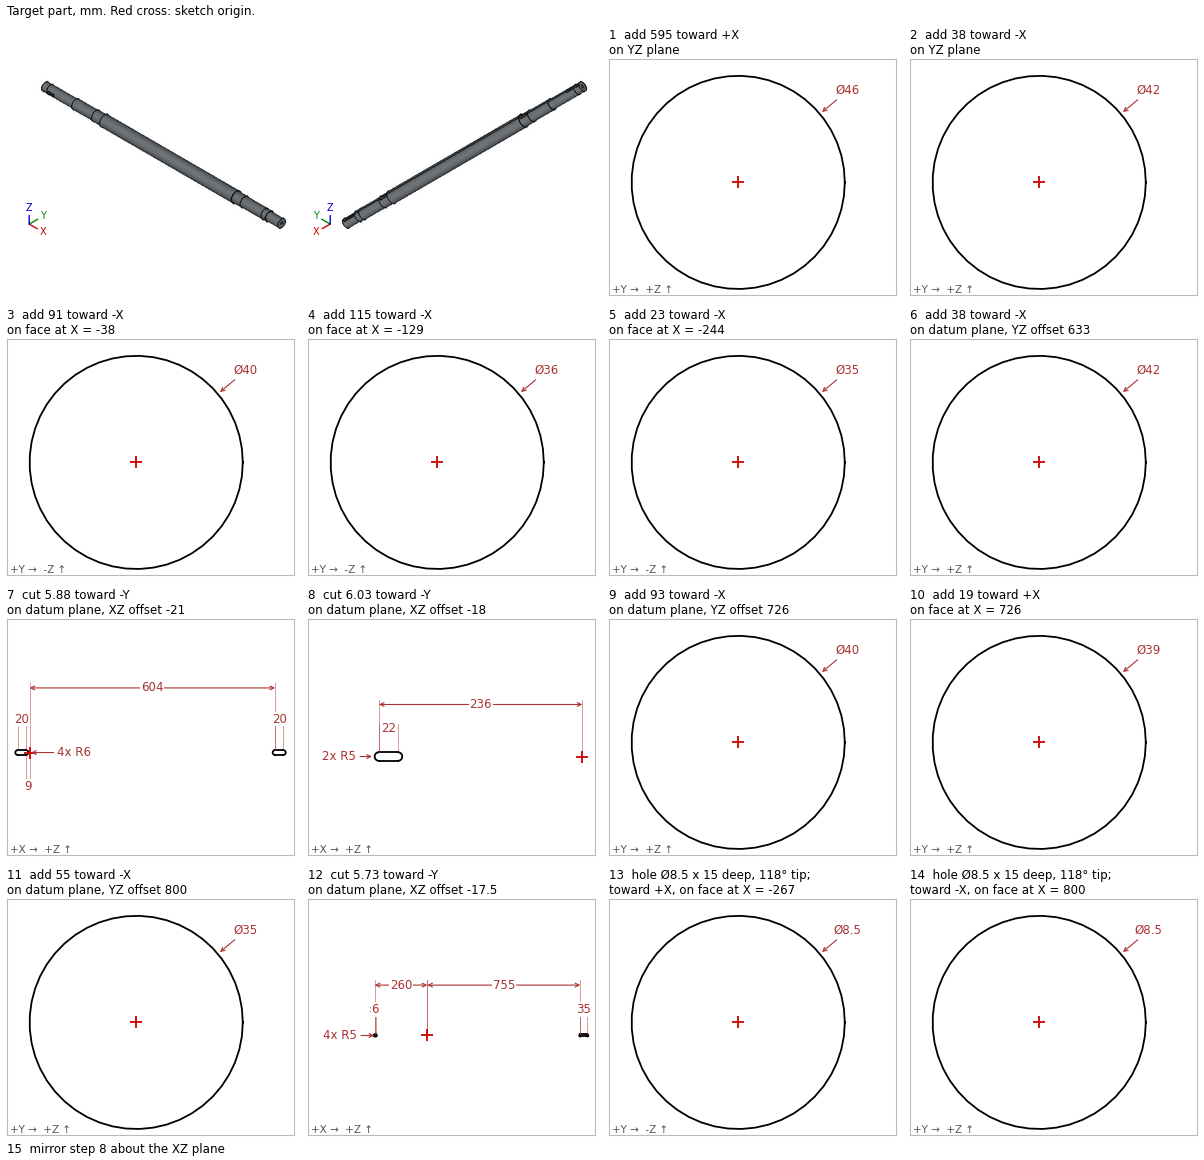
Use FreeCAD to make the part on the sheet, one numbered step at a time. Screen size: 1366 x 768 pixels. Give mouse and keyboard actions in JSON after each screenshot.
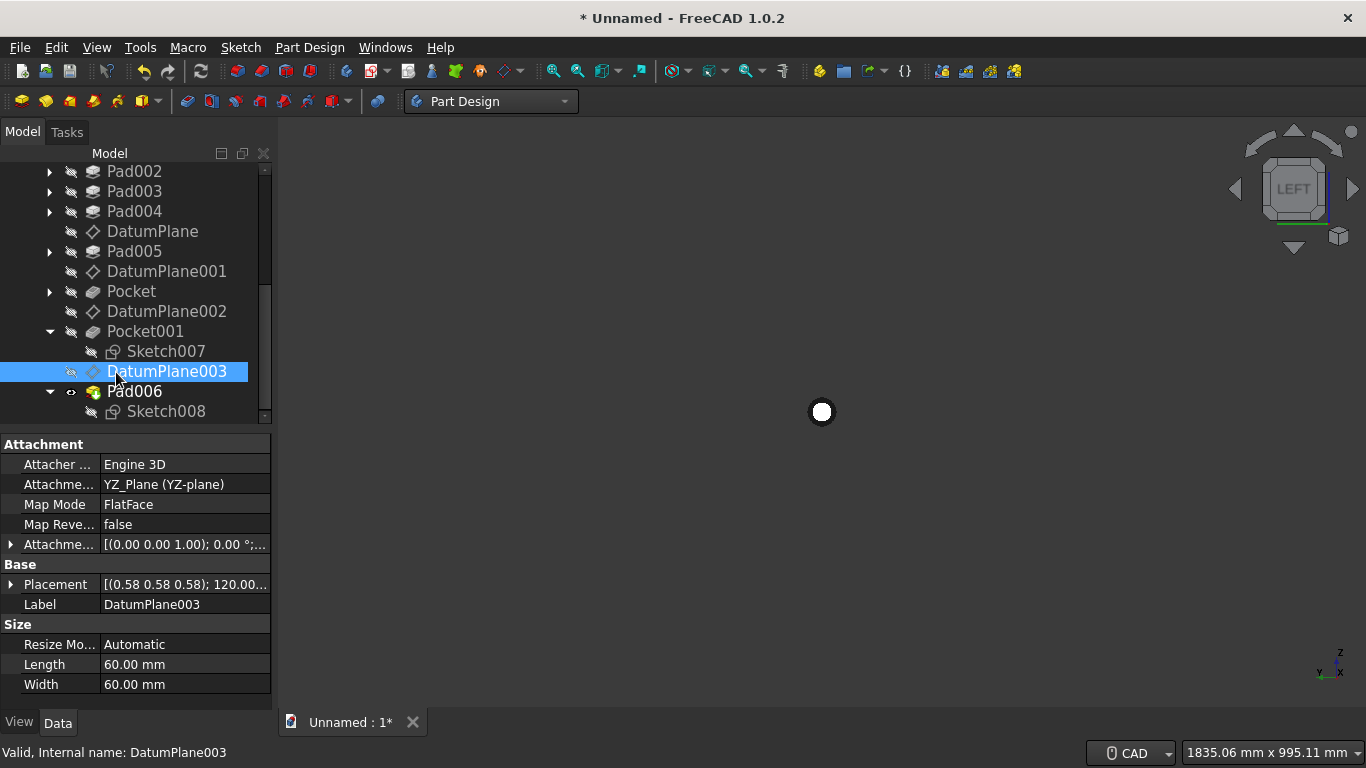
{"action": "key", "text": "0"}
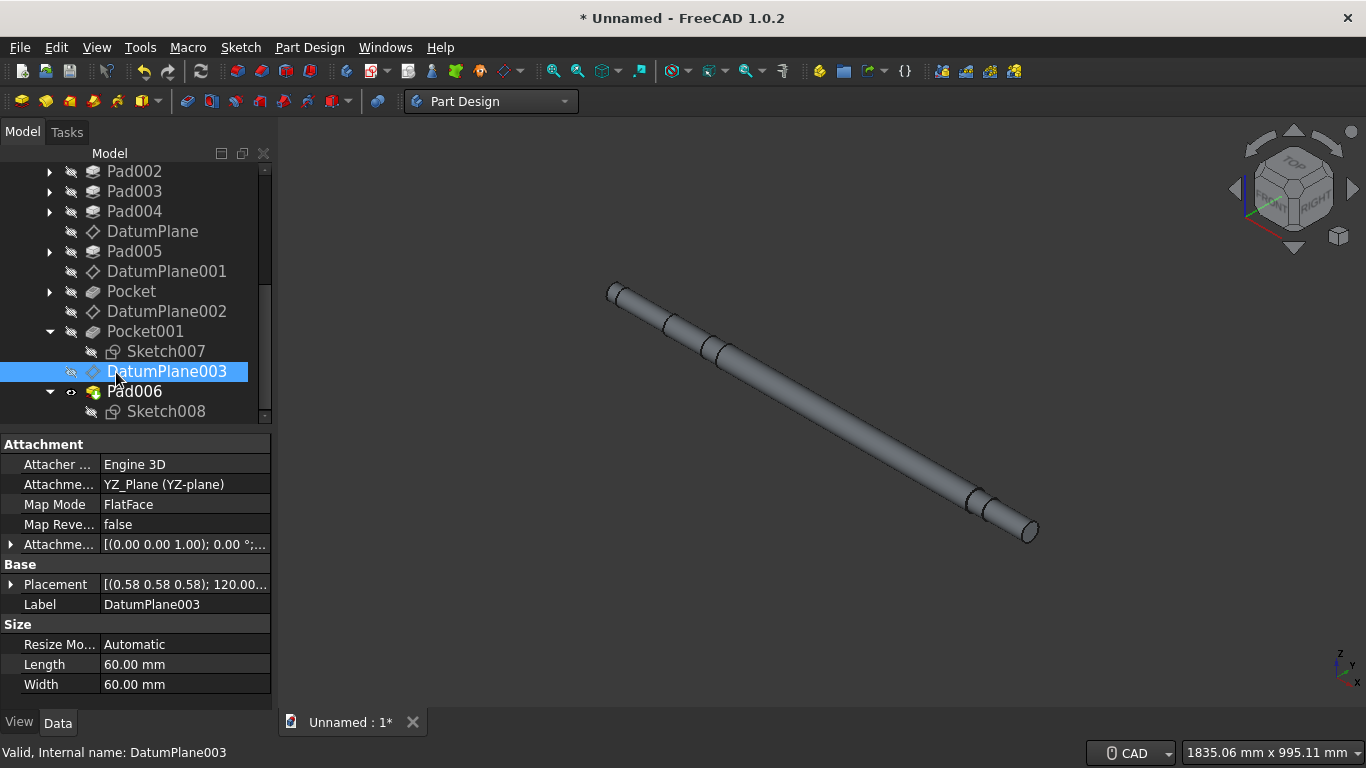
{"action": "key", "text": "3"}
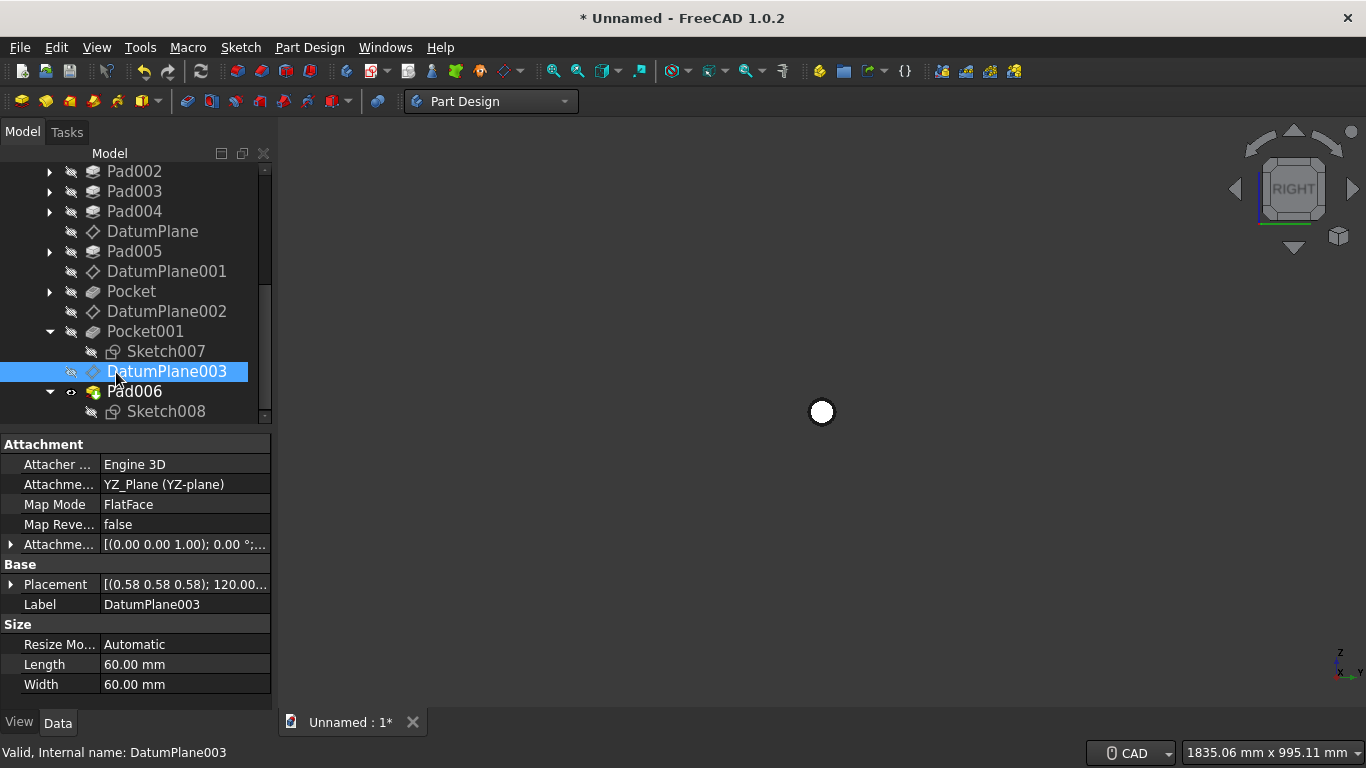
{"action": "left_click", "coordinate": [554, 72]}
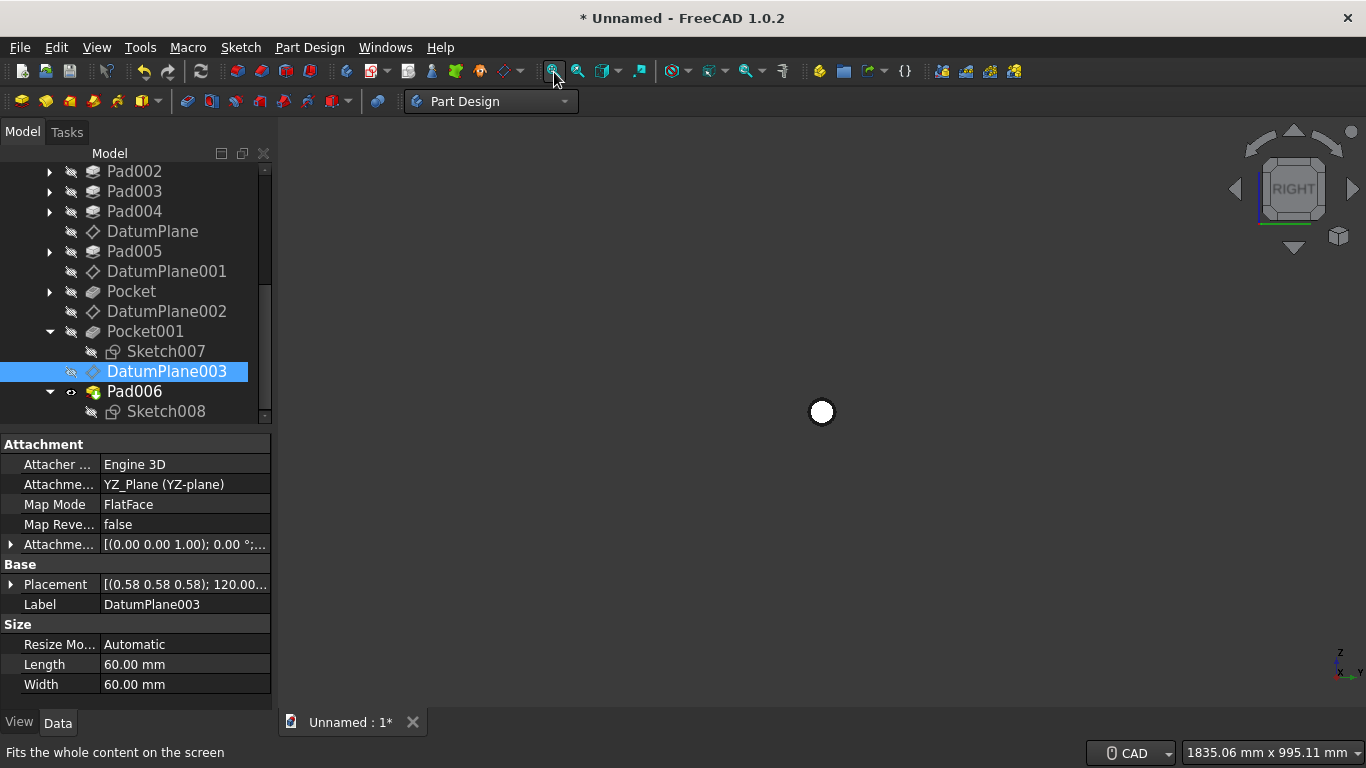
{"action": "left_click", "coordinate": [822, 411]}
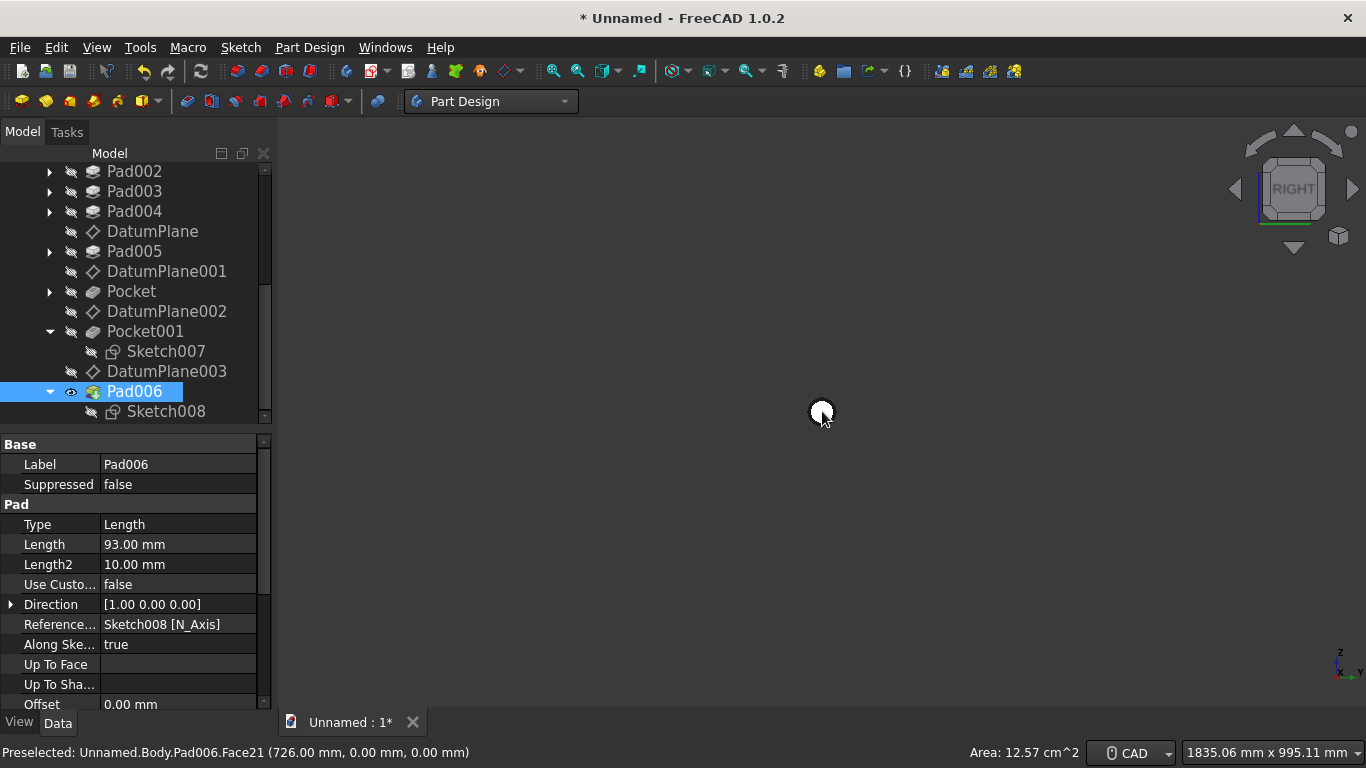
{"action": "left_click", "coordinate": [372, 72]}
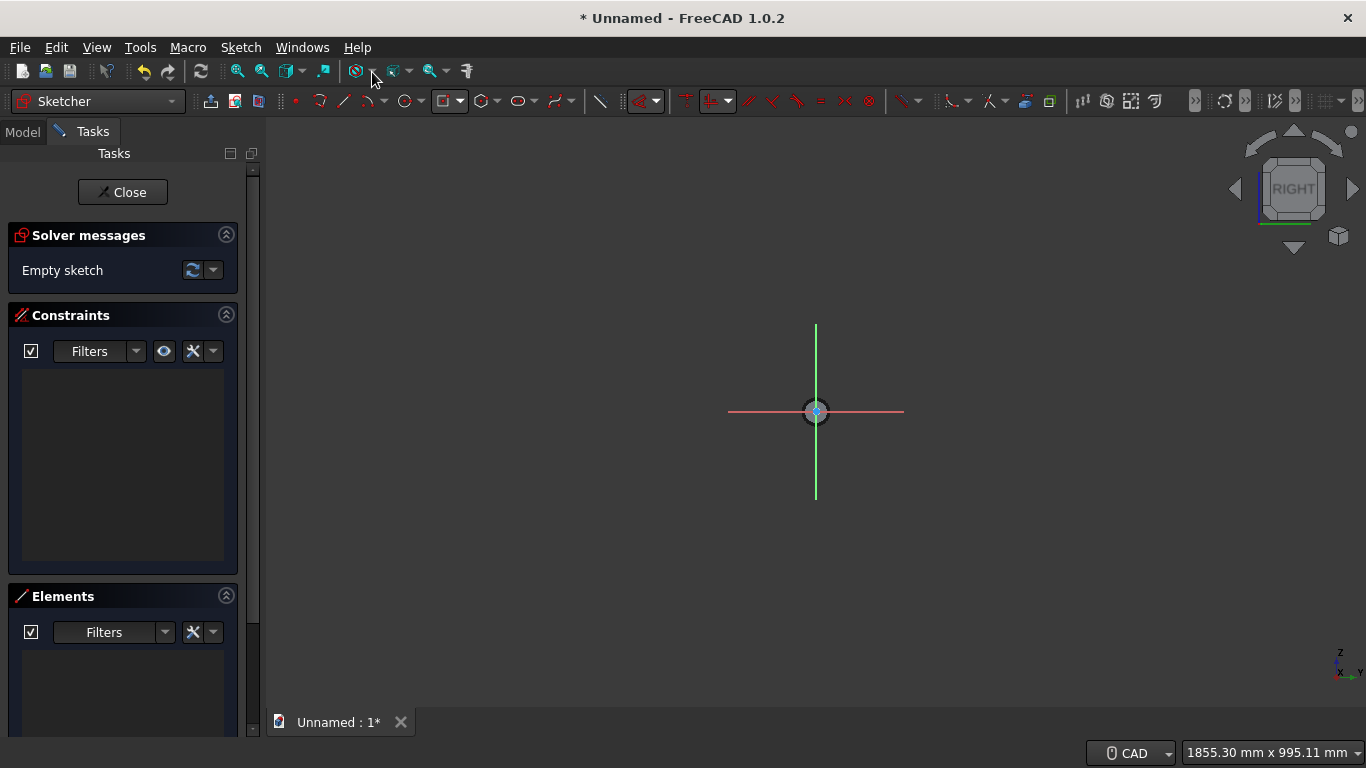
{"action": "scroll", "coordinate": [820, 412], "scroll_direction": "up", "scroll_amount": 14}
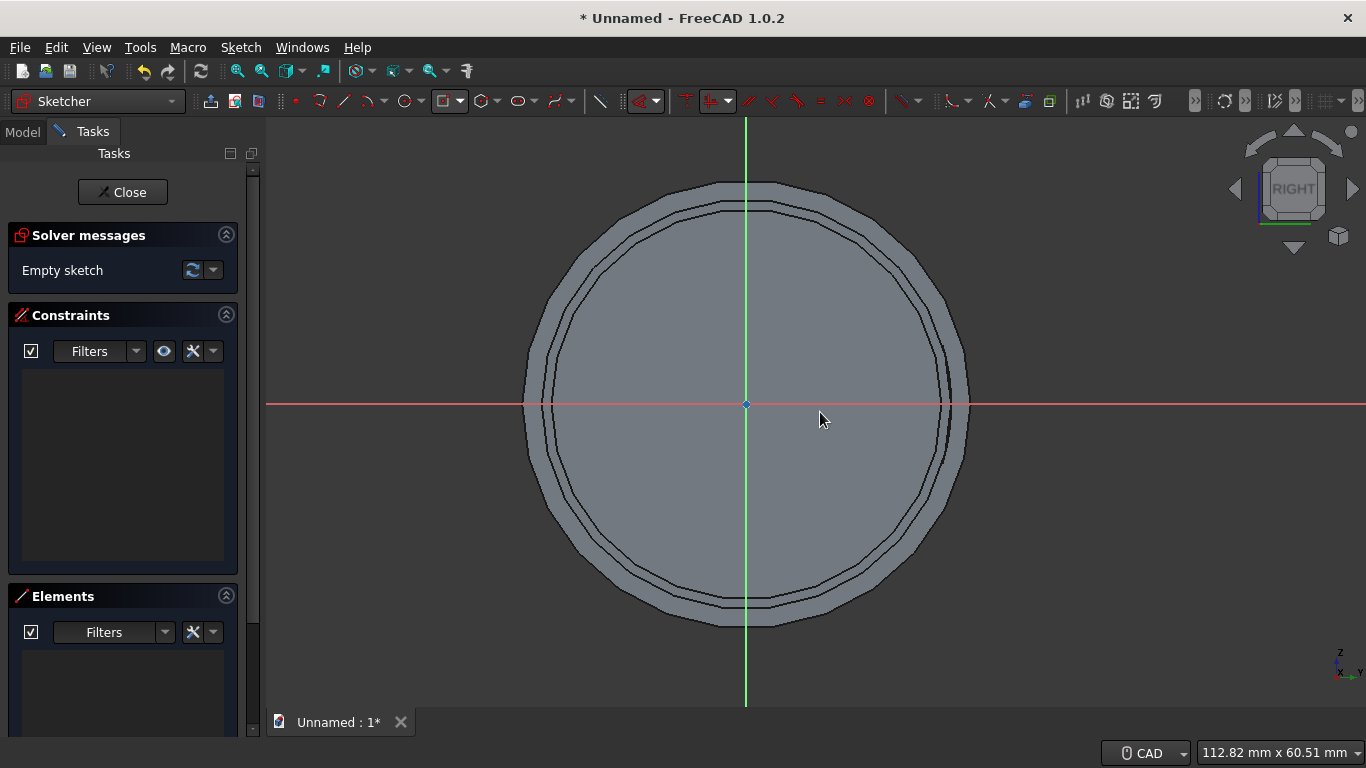
{"action": "key", "text": "g c"}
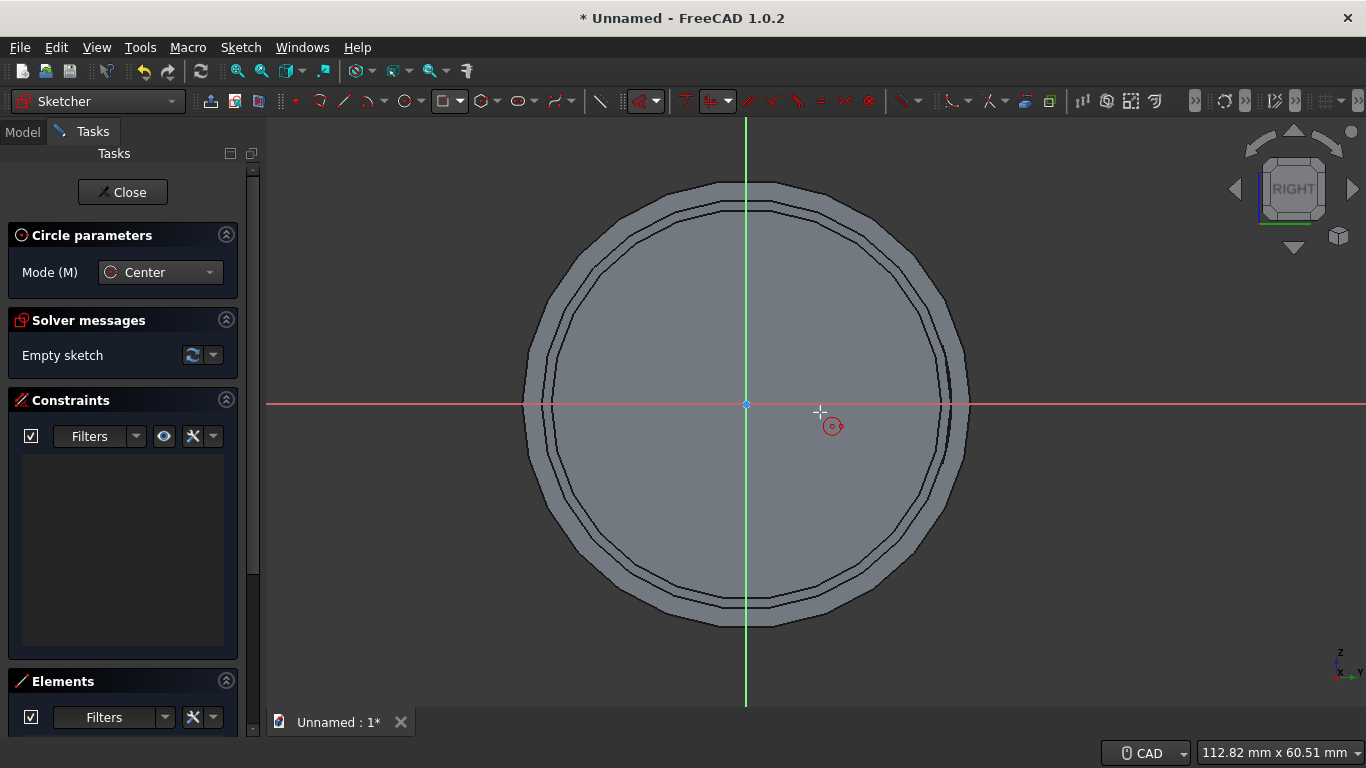
{"action": "left_click", "coordinate": [746, 404]}
{"action": "mouse_move", "coordinate": [881, 270]}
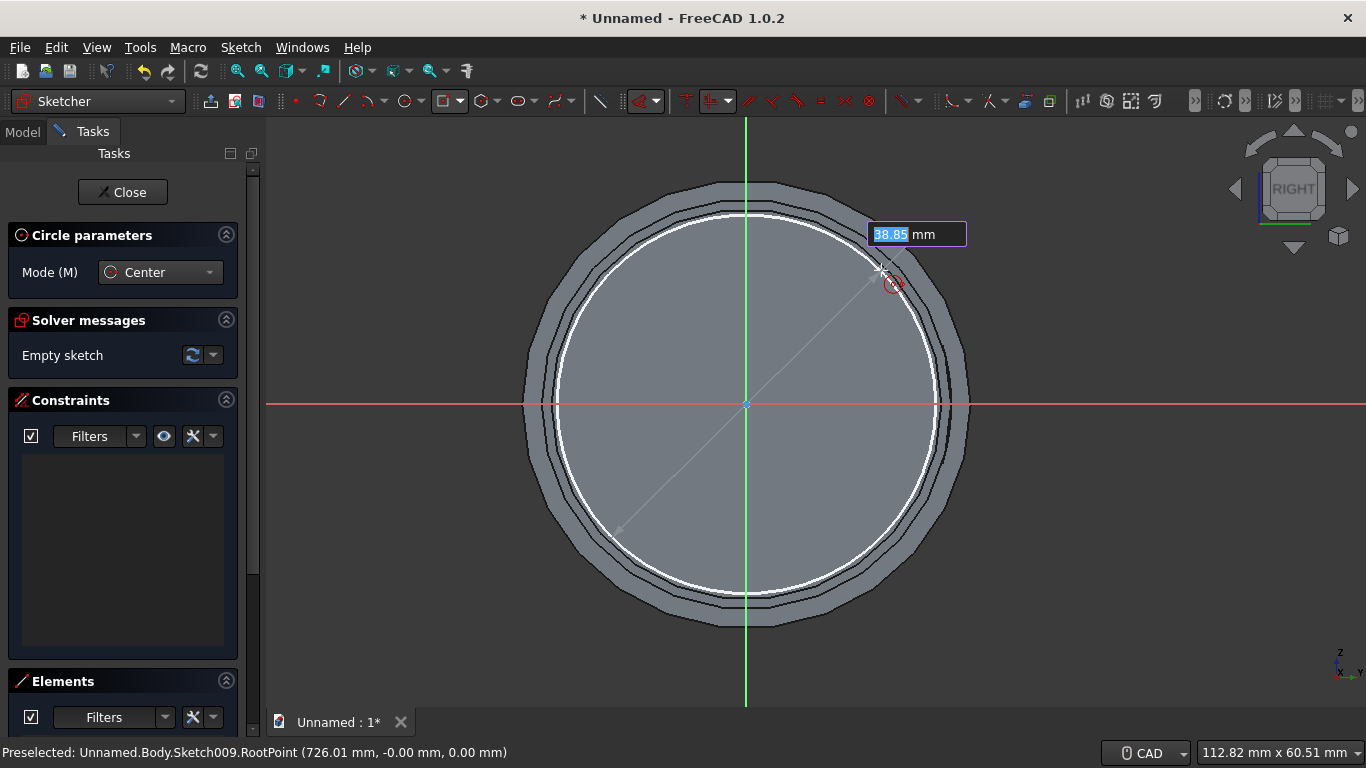
{"action": "type", "text": "39"}
{"action": "key", "text": "Return"}
{"action": "key", "text": "Escape"}